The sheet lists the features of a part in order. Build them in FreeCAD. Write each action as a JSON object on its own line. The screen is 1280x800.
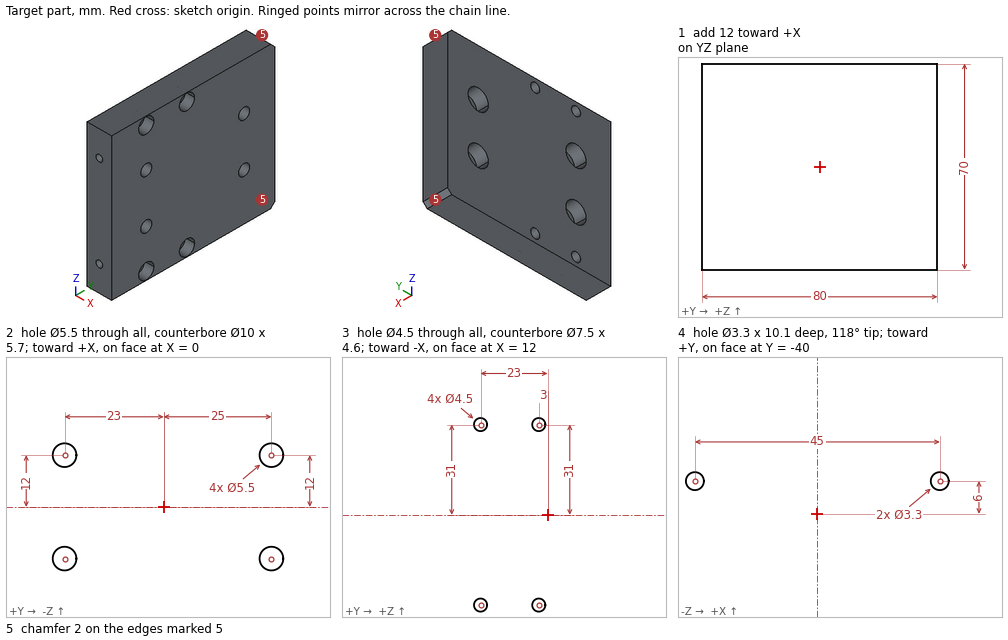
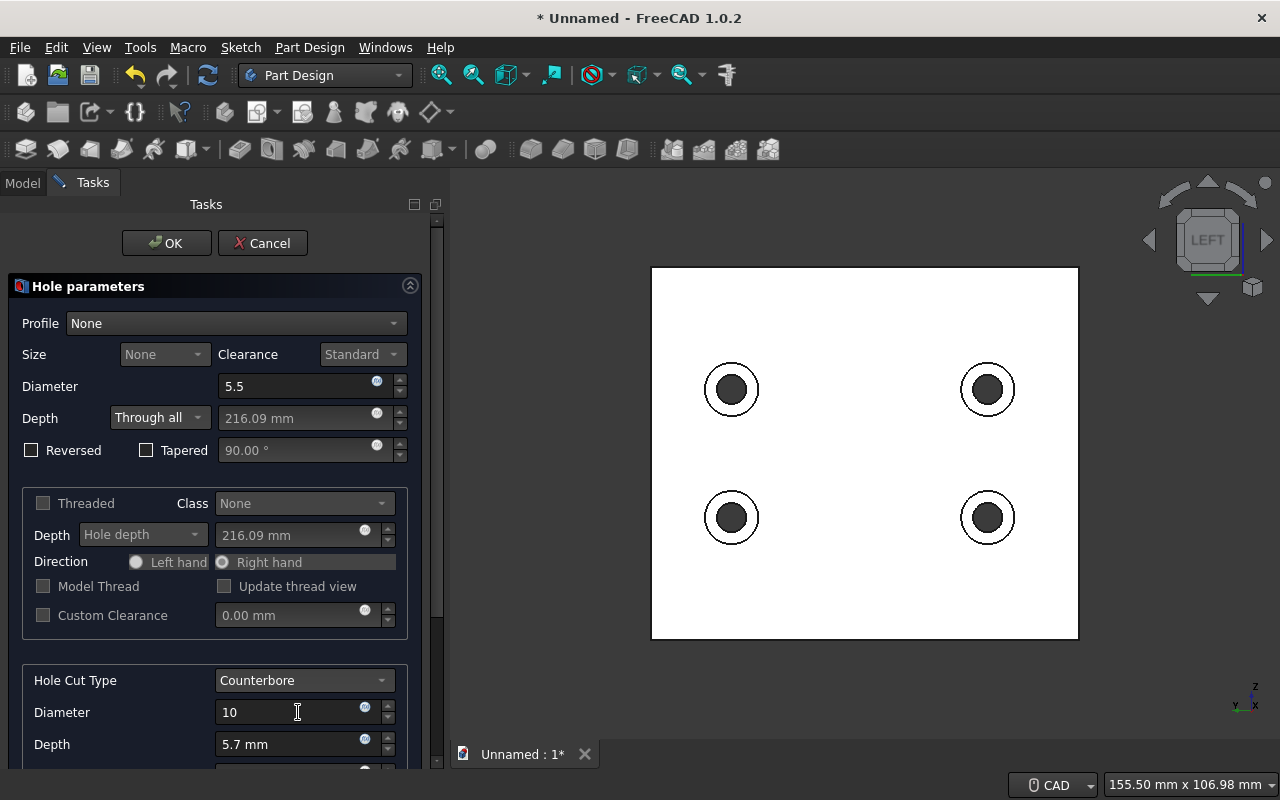
{"action": "left_click", "coordinate": [167, 243]}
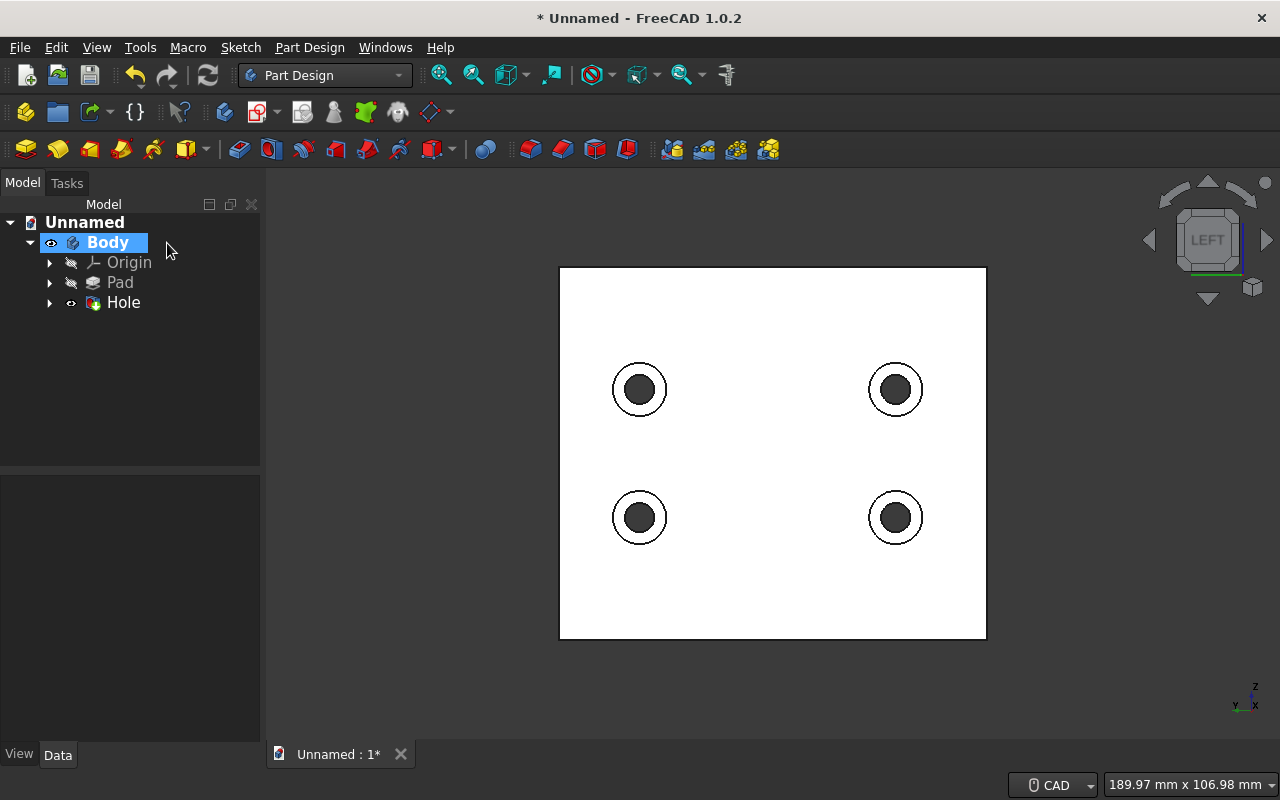
{"action": "key", "text": "0"}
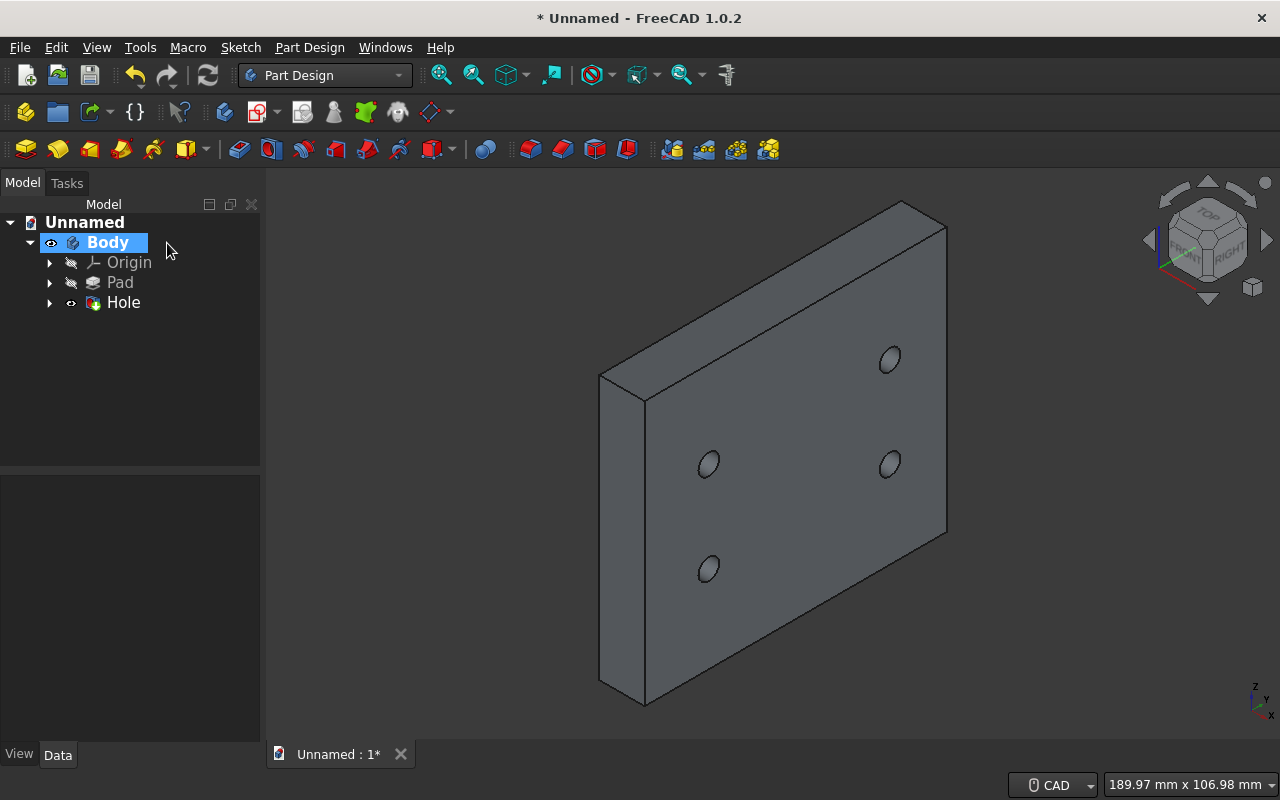
{"action": "left_click", "coordinate": [796, 466]}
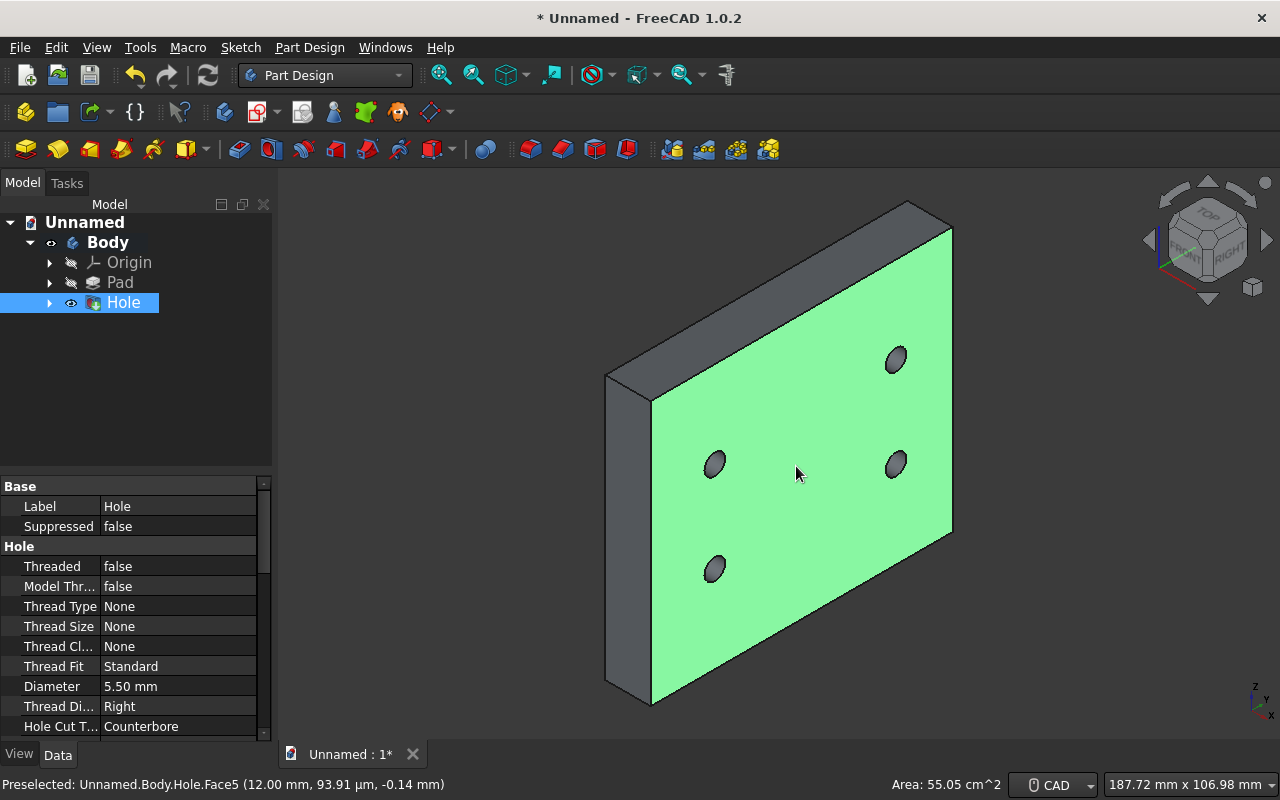
{"action": "left_click", "coordinate": [258, 112]}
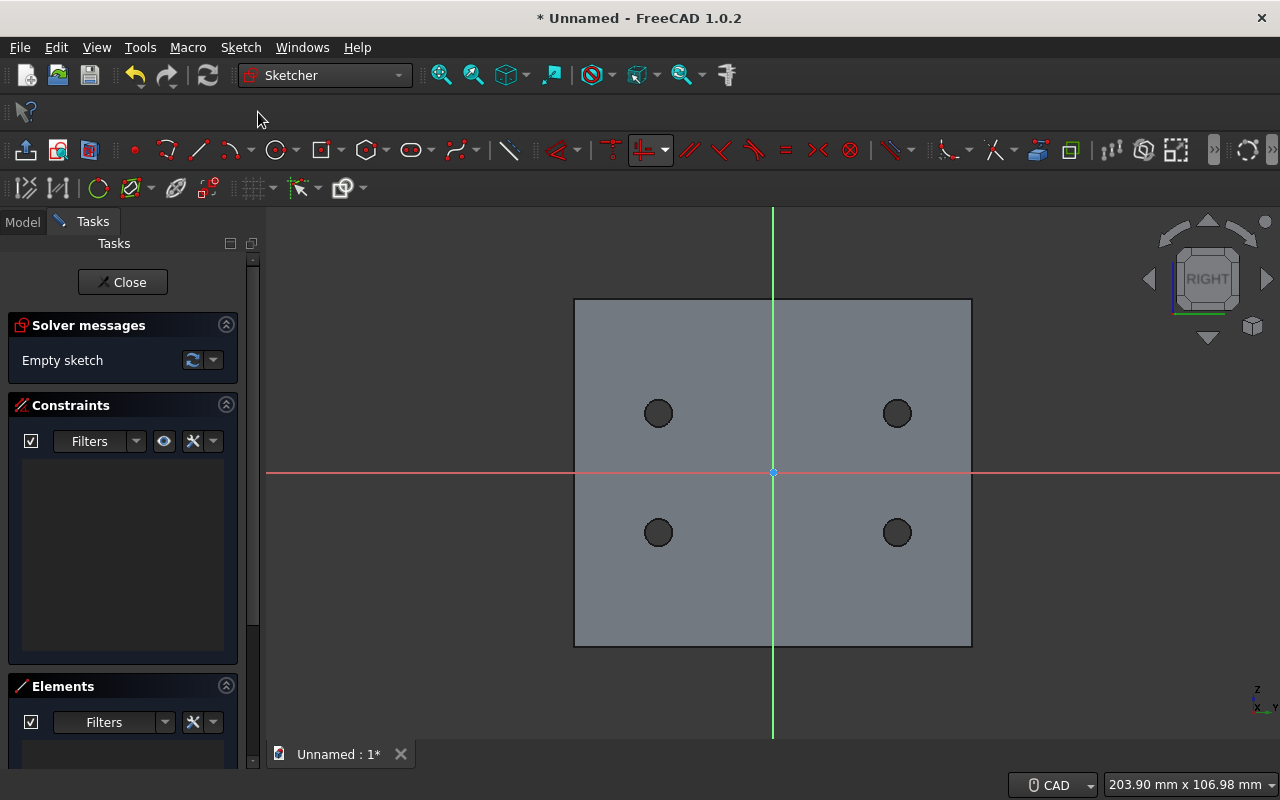
{"action": "left_click", "coordinate": [276, 150]}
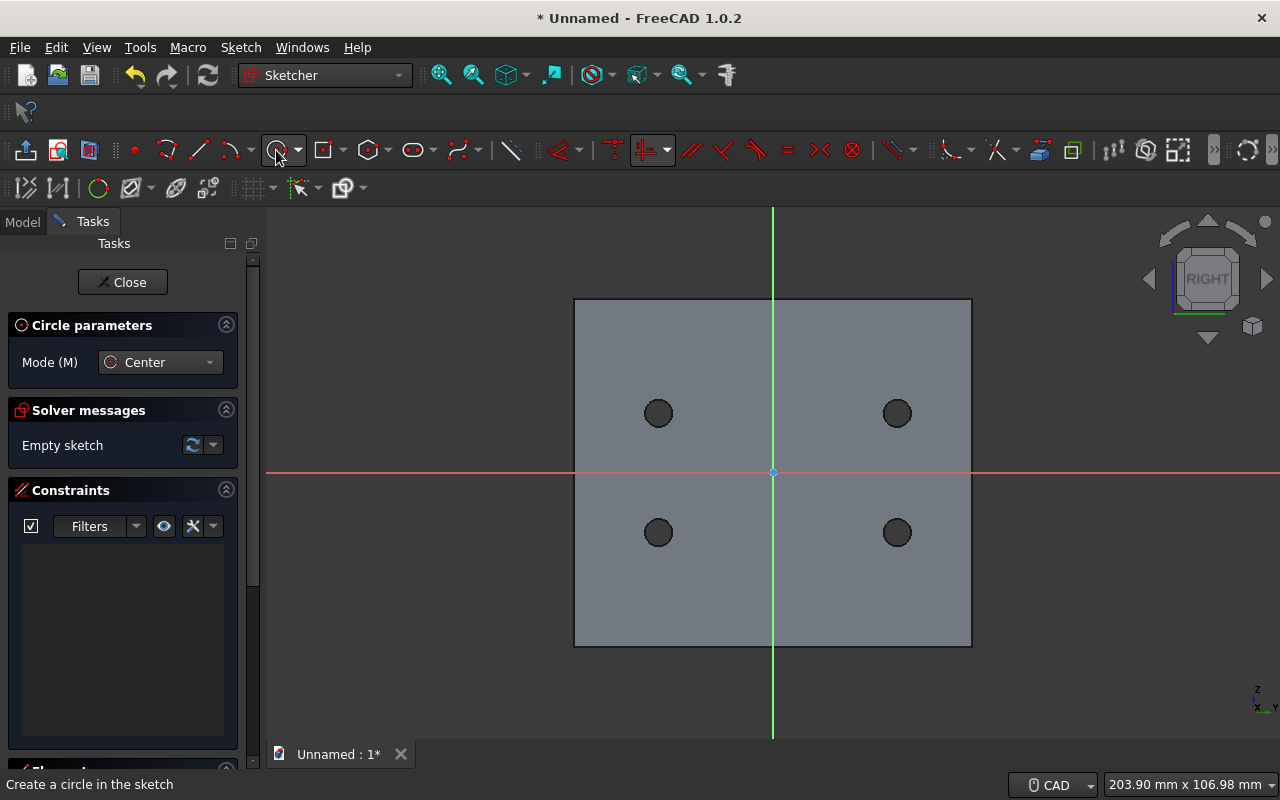
{"action": "scroll", "coordinate": [659, 319], "scroll_direction": "up", "scroll_amount": 4}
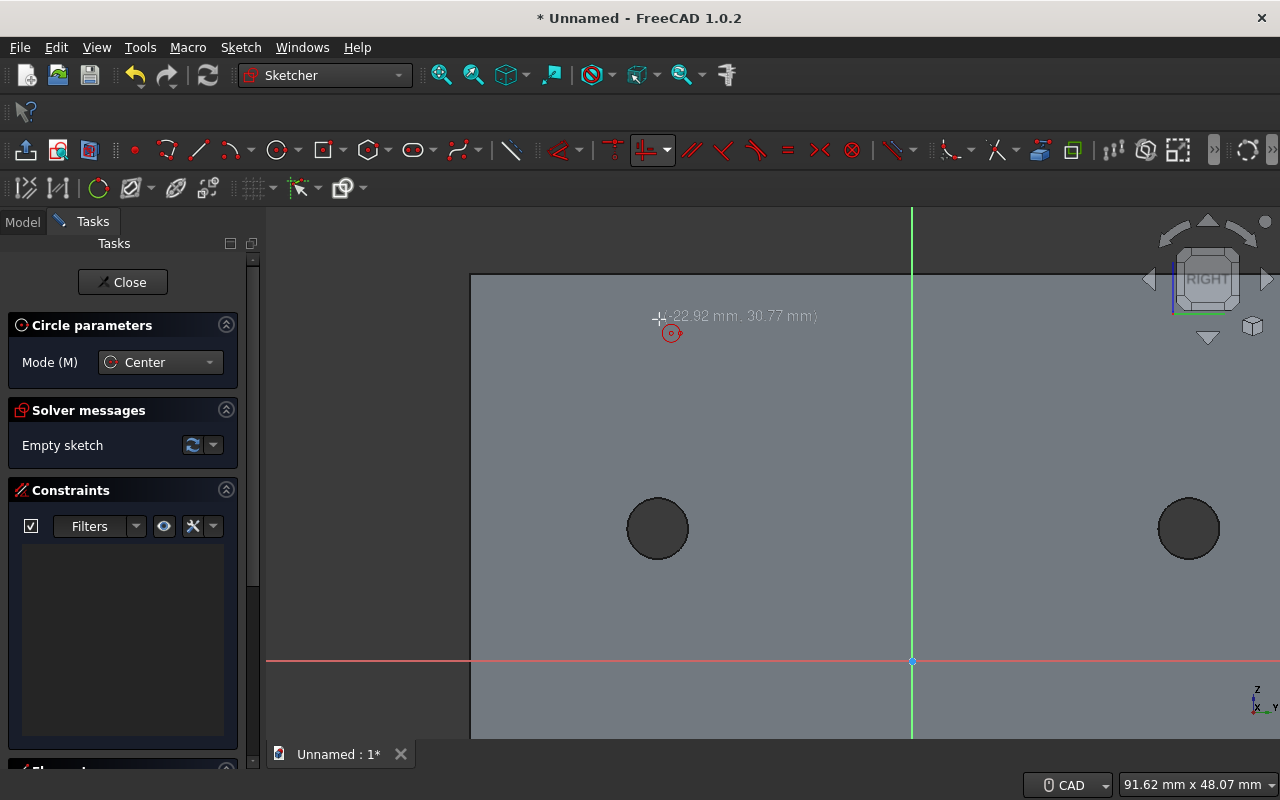
{"action": "left_click", "coordinate": [658, 318]}
{"action": "left_click", "coordinate": [675, 301]}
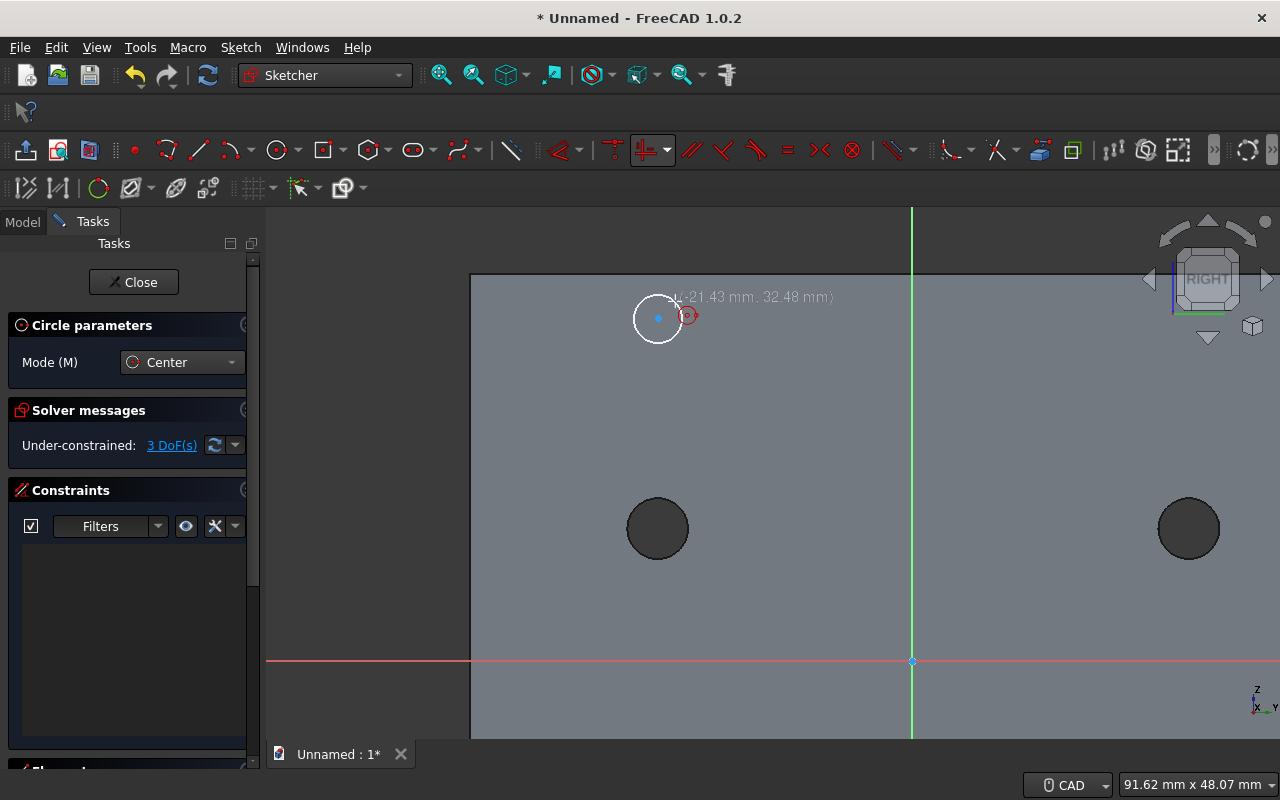
{"action": "left_click", "coordinate": [879, 318]}
{"action": "left_click", "coordinate": [897, 301]}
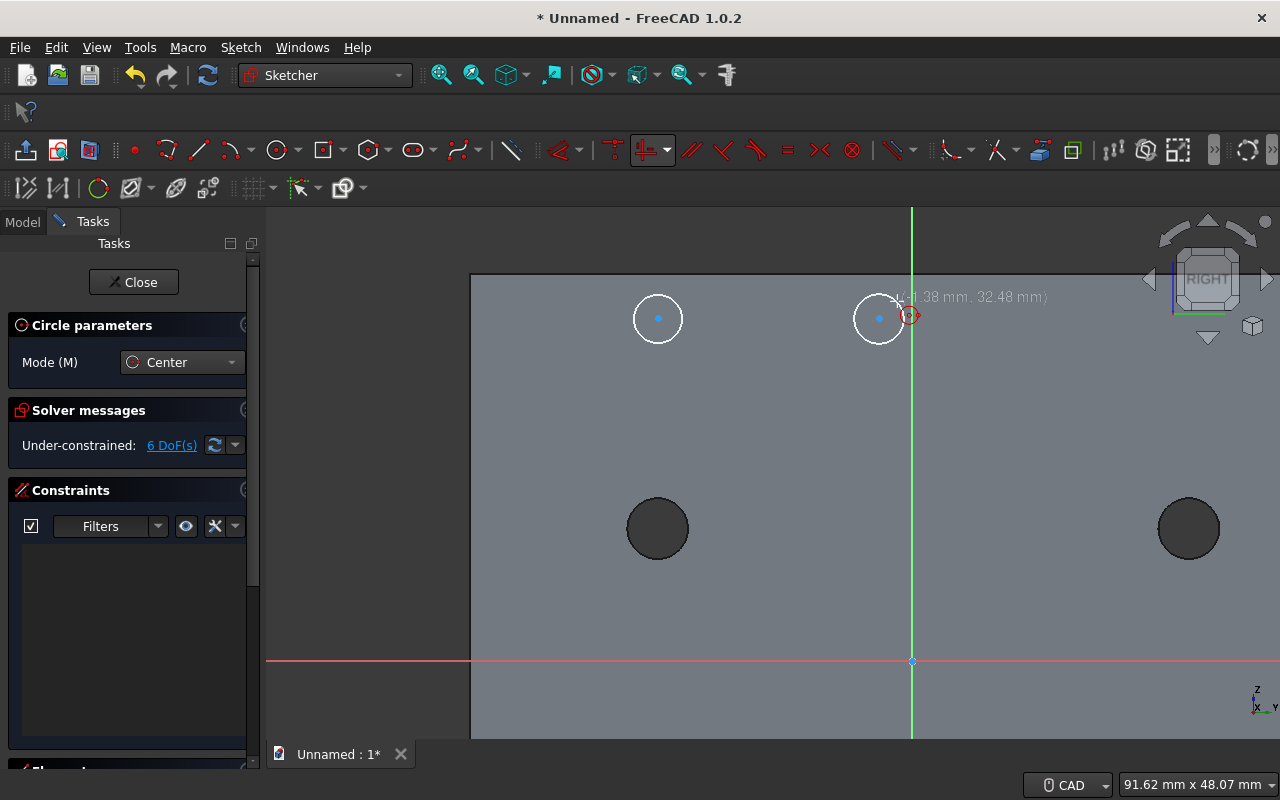
{"action": "scroll", "coordinate": [649, 319], "scroll_direction": "down", "scroll_amount": 4}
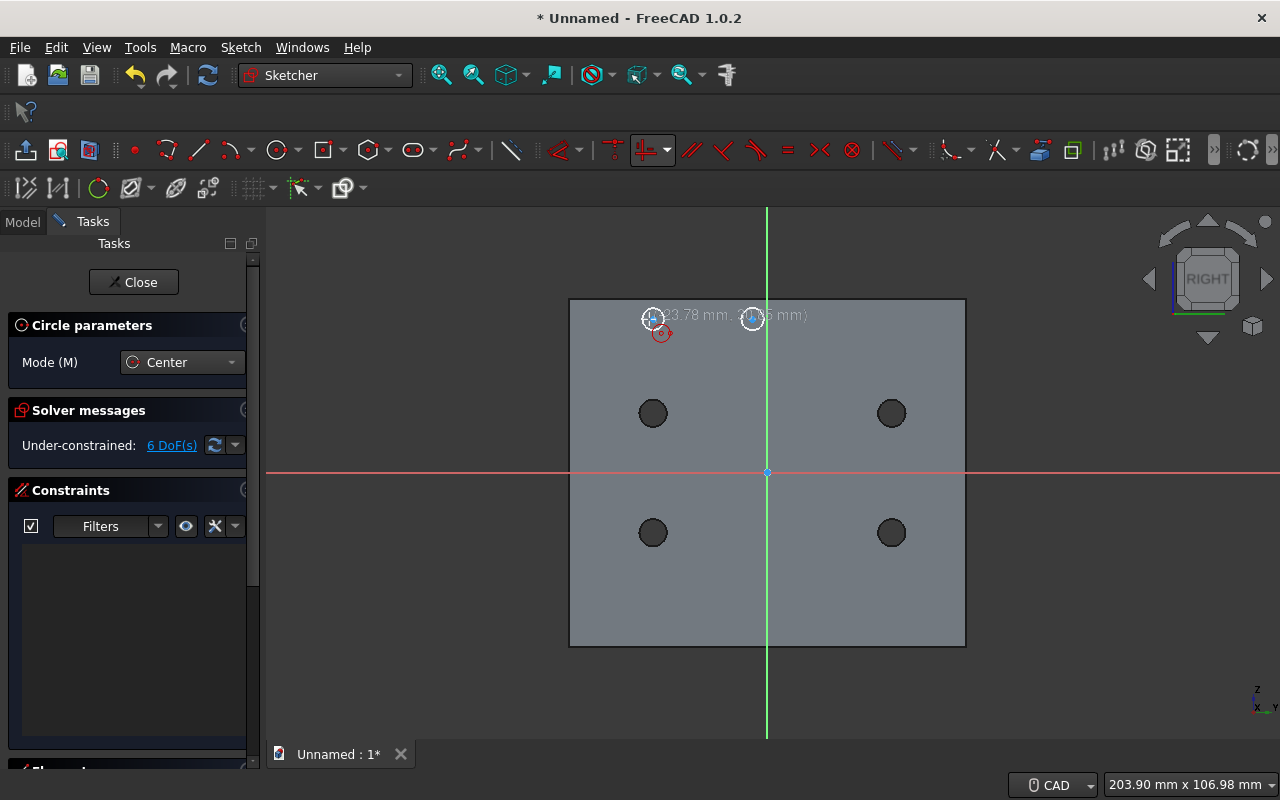
{"action": "scroll", "coordinate": [753, 627], "scroll_direction": "up", "scroll_amount": 4}